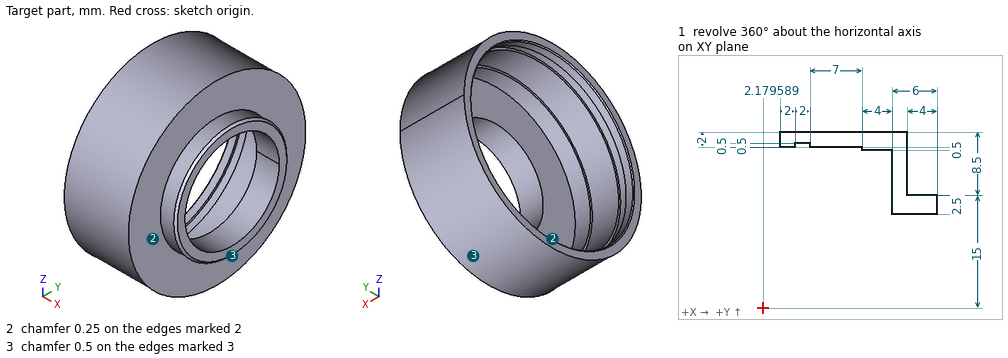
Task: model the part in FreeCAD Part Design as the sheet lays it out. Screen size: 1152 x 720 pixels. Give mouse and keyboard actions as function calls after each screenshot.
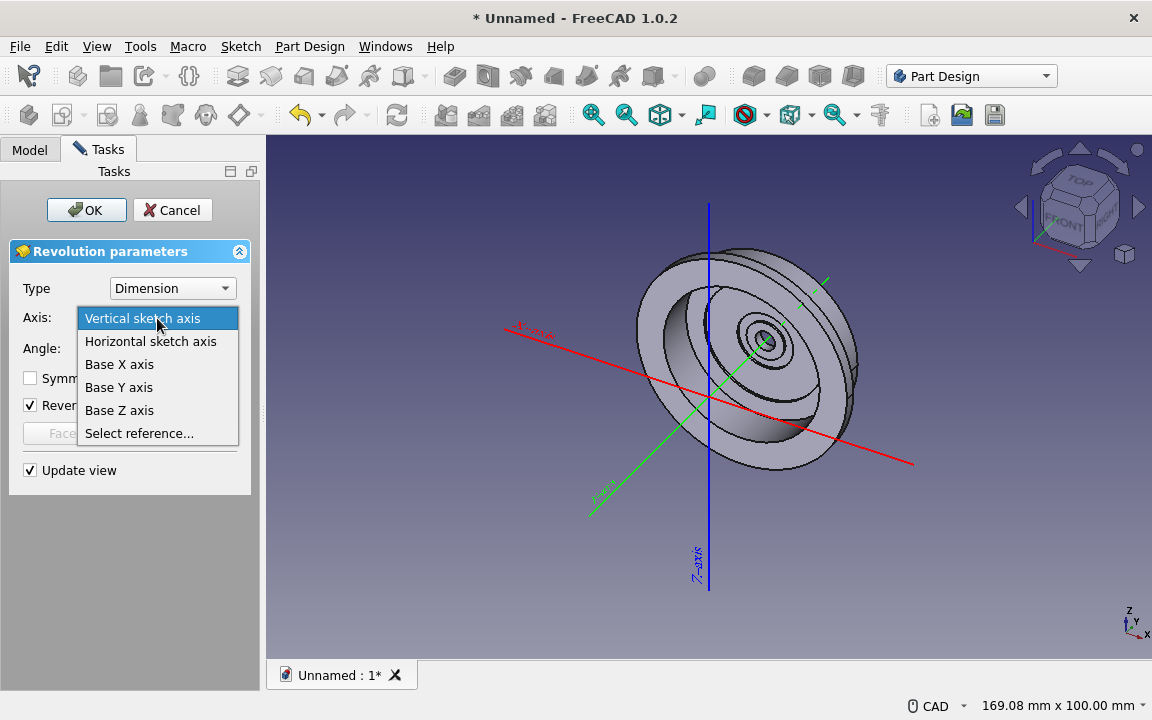
click(156, 342)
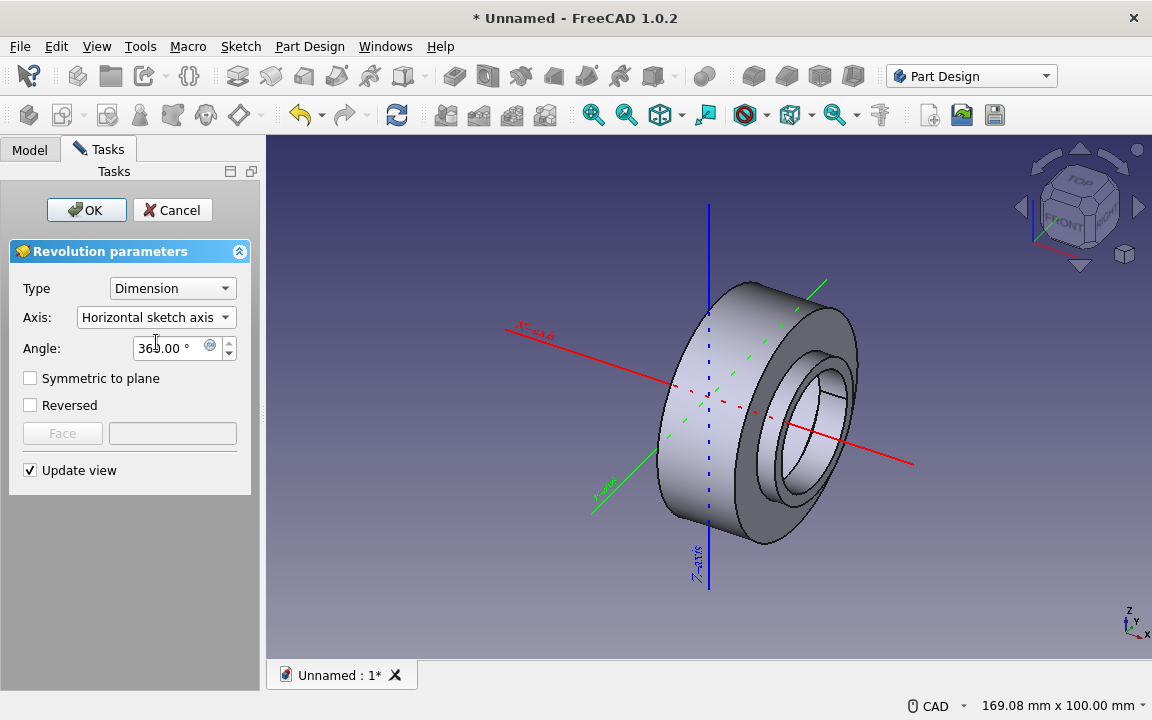
click(87, 210)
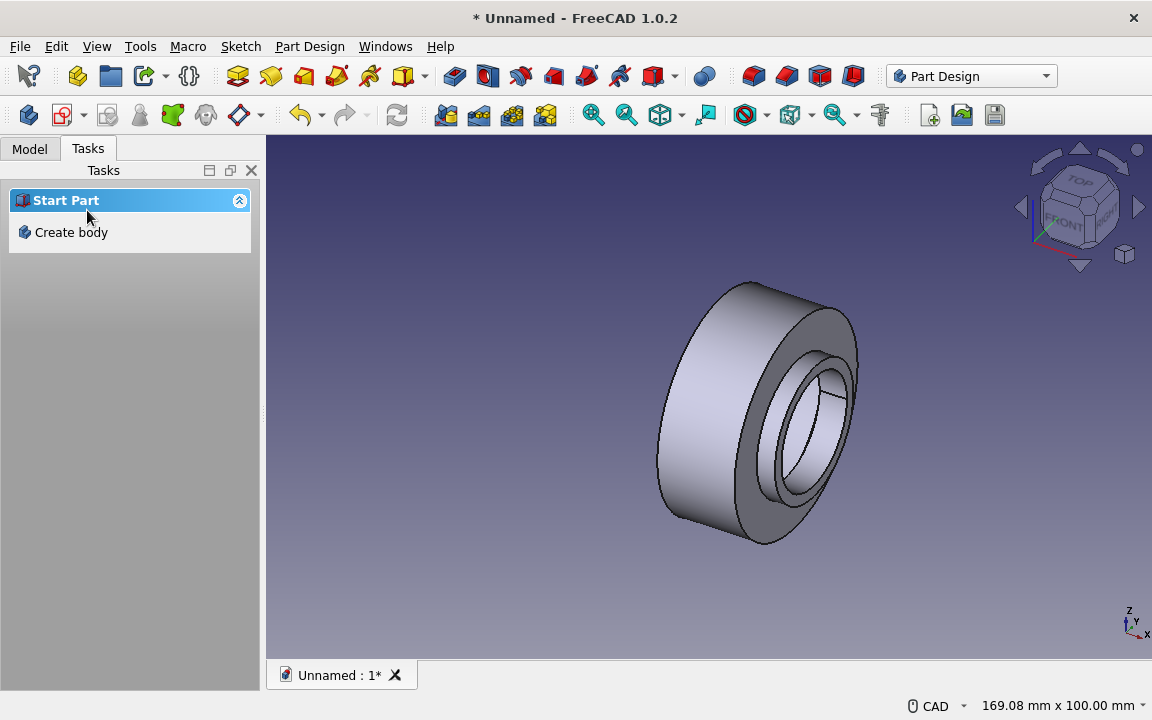
key(0)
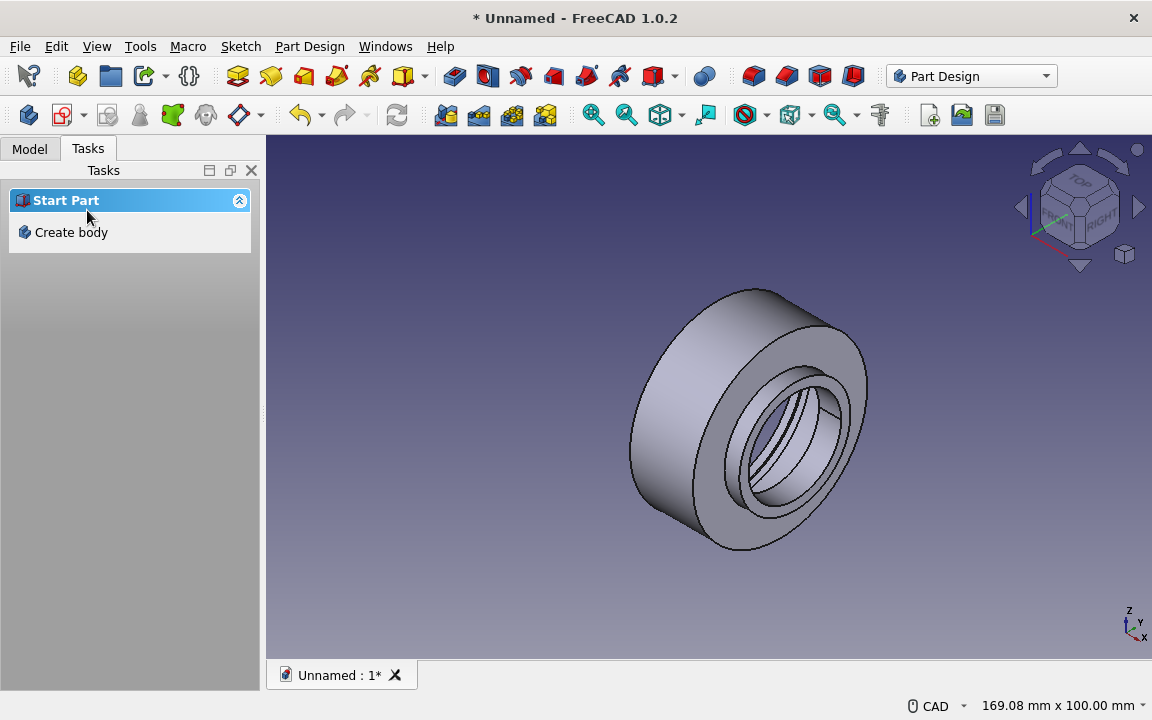
key(2)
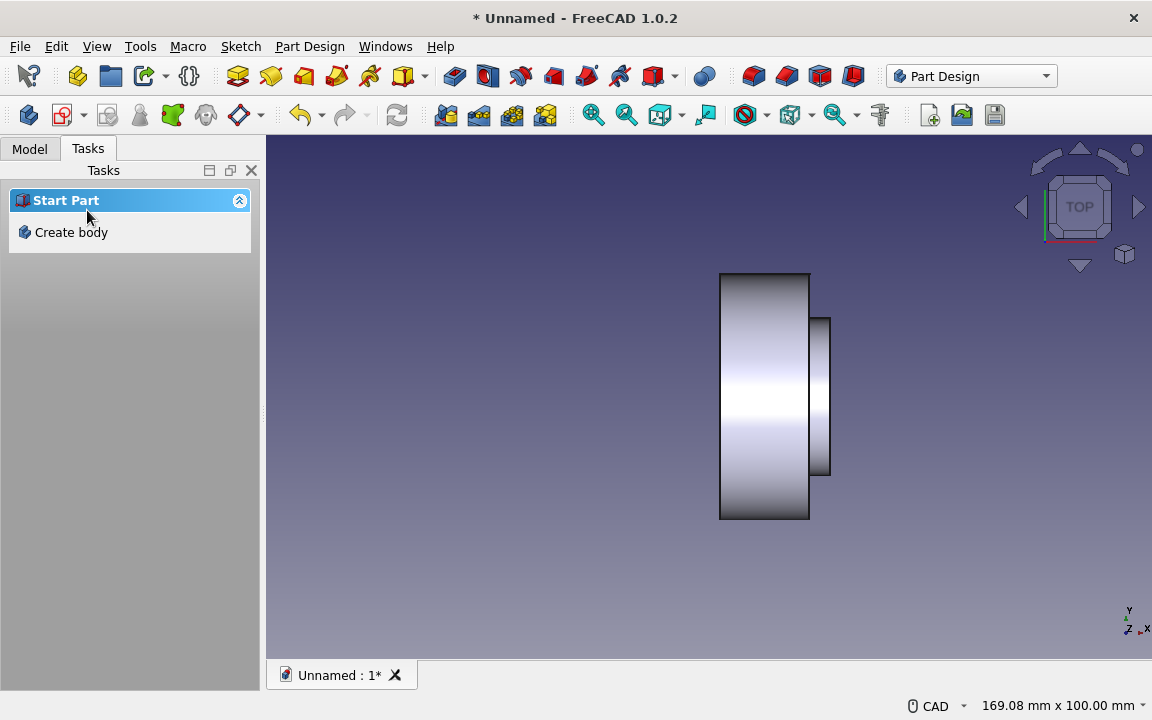
key(1)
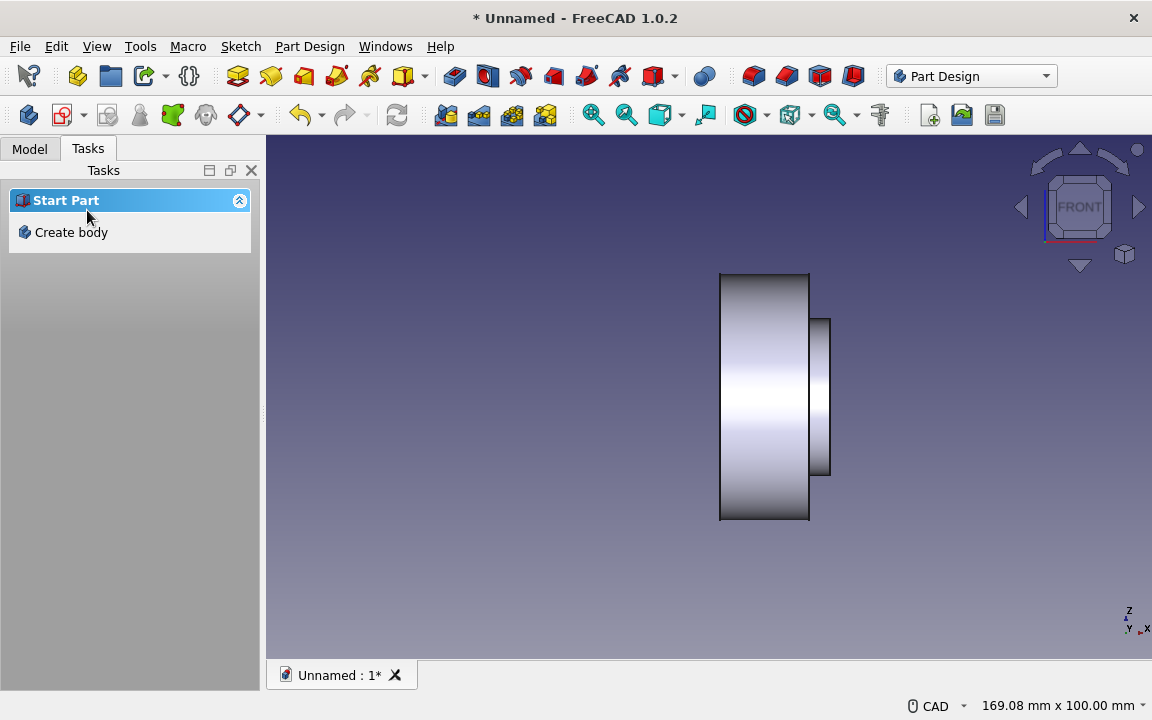
key(3)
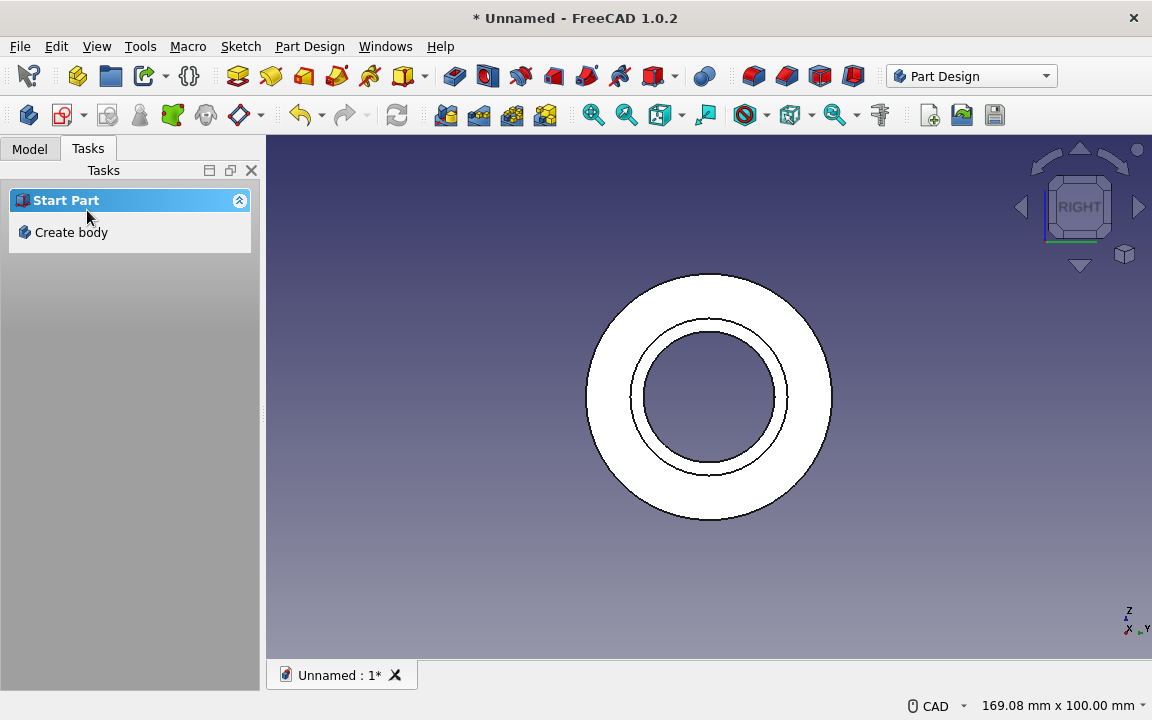
key(5)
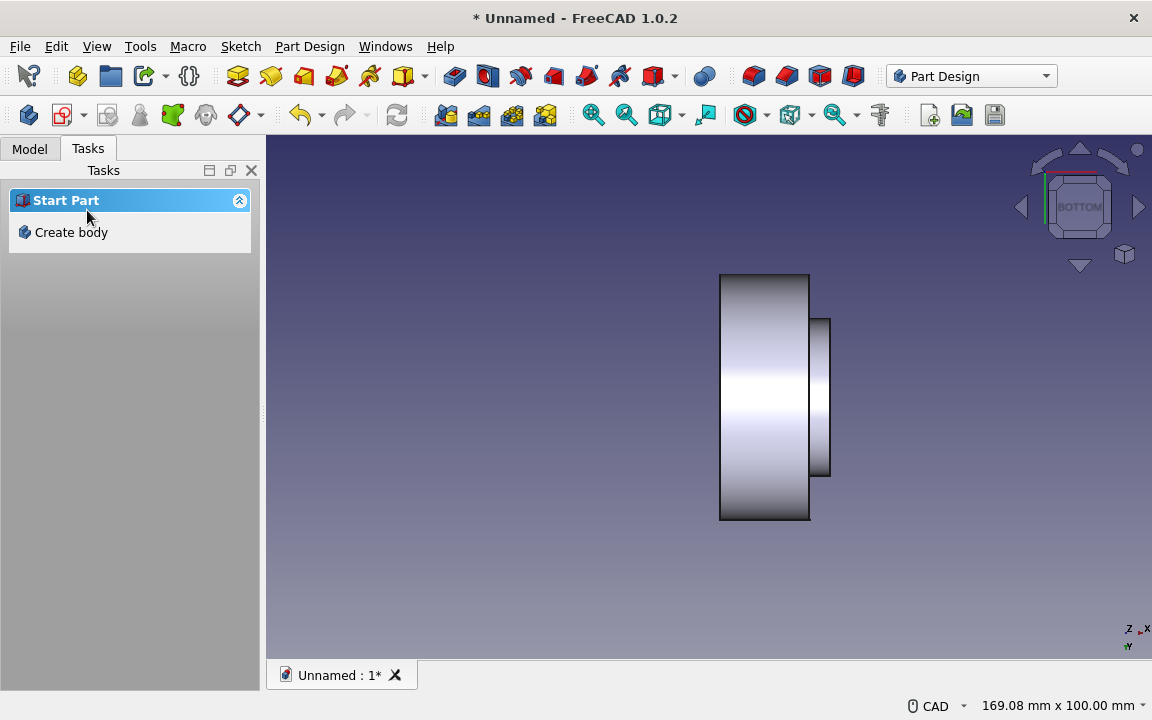
key(4)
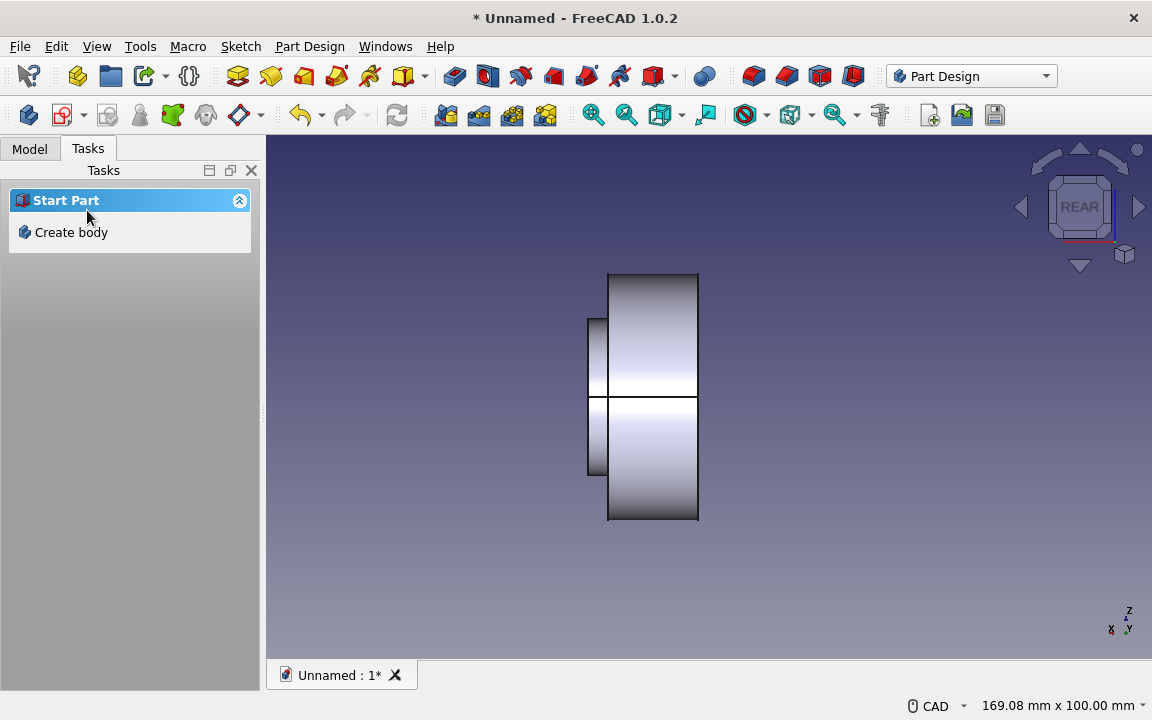
key(6)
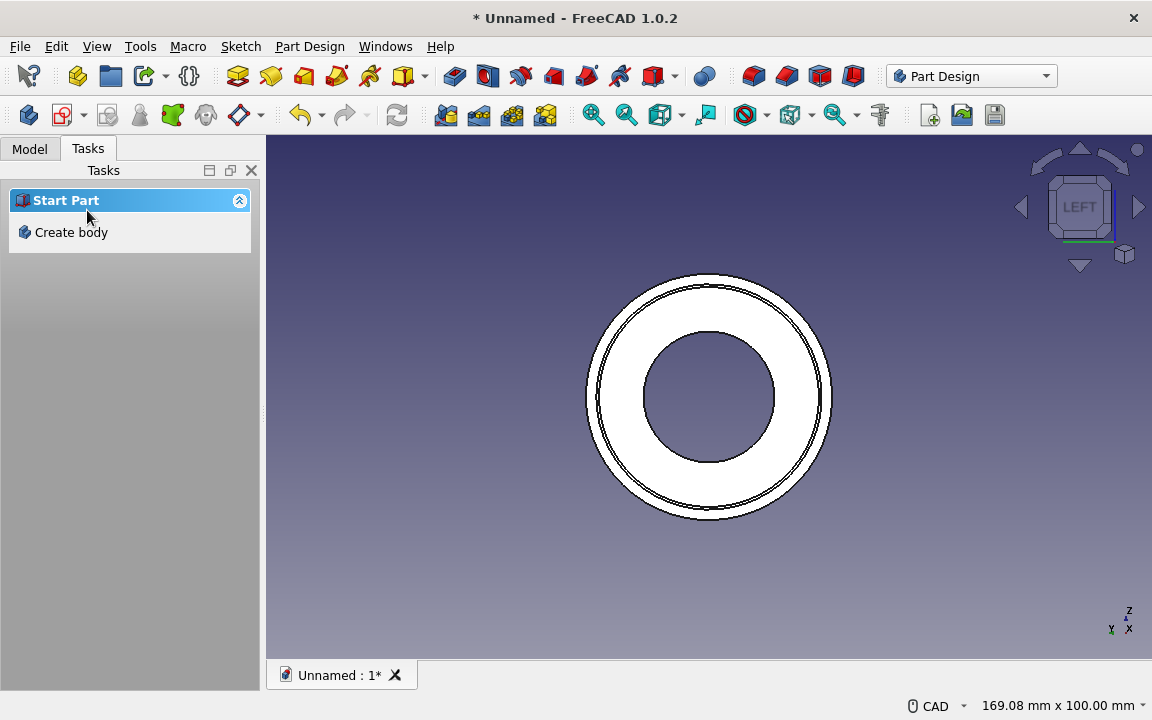
click(822, 396)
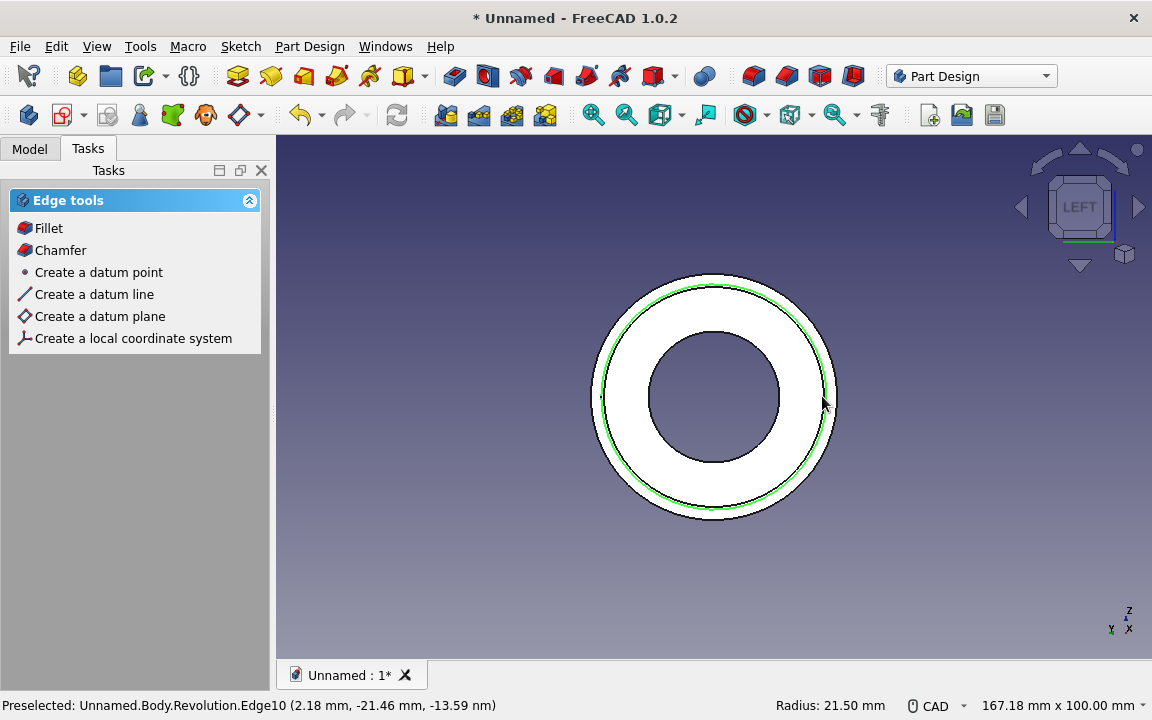
click(787, 76)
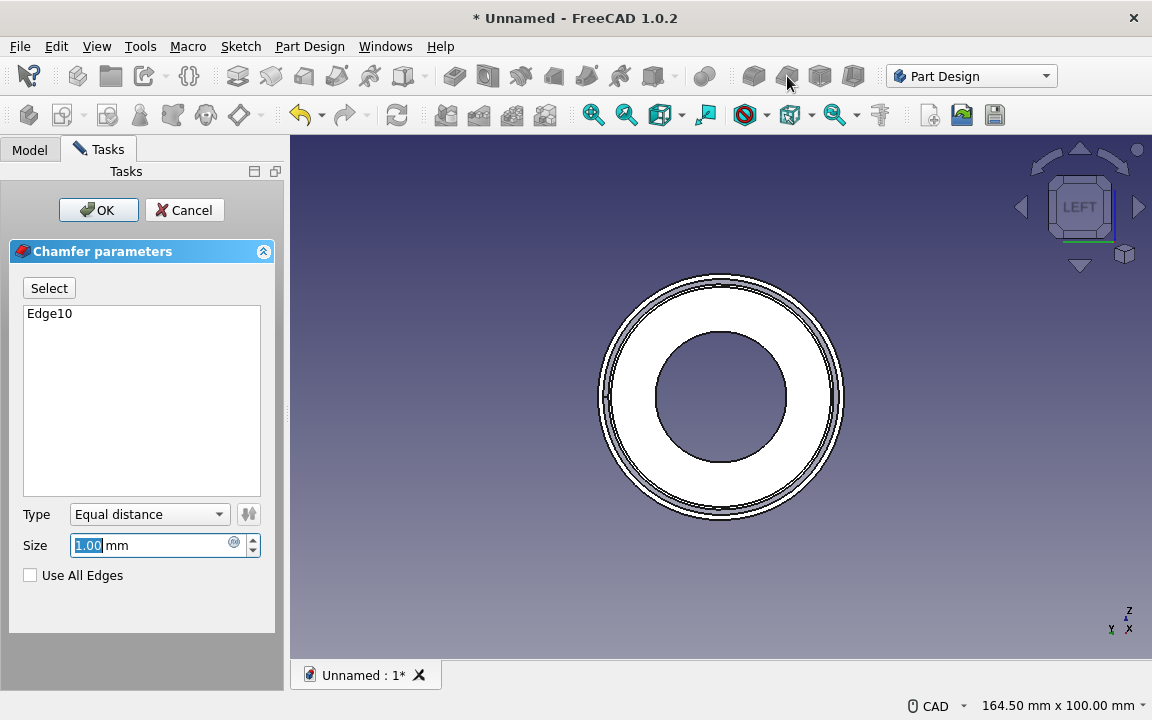
text(0.25)
key(Tab)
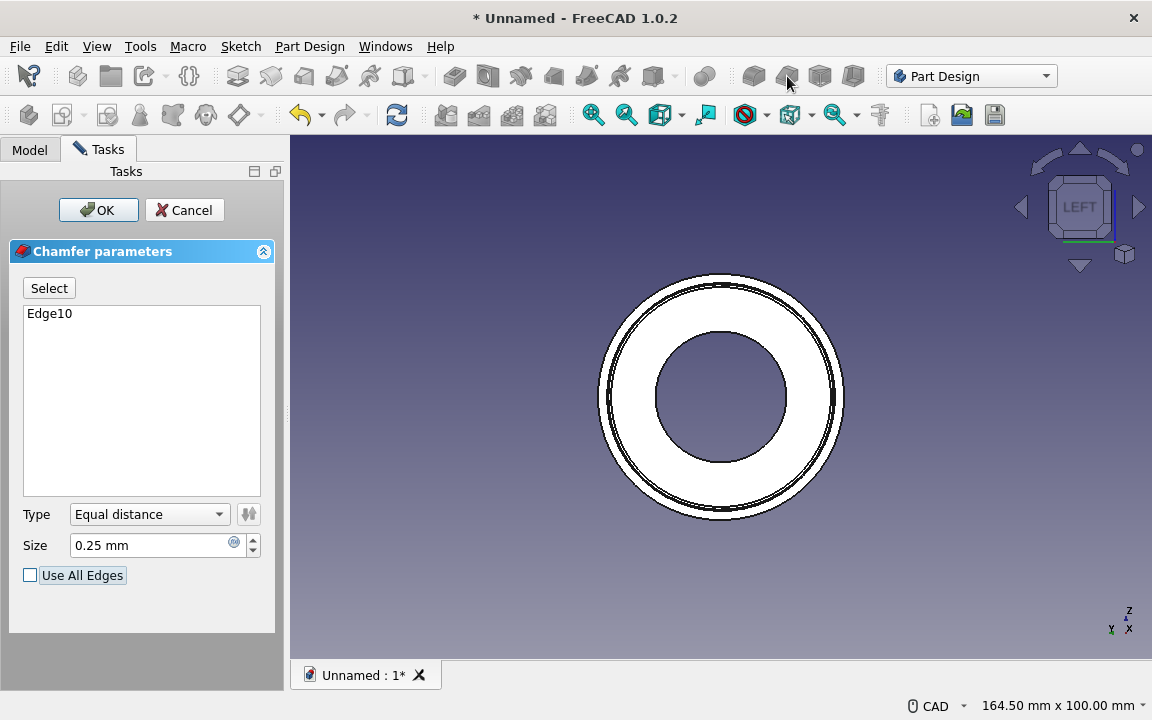
click(99, 210)